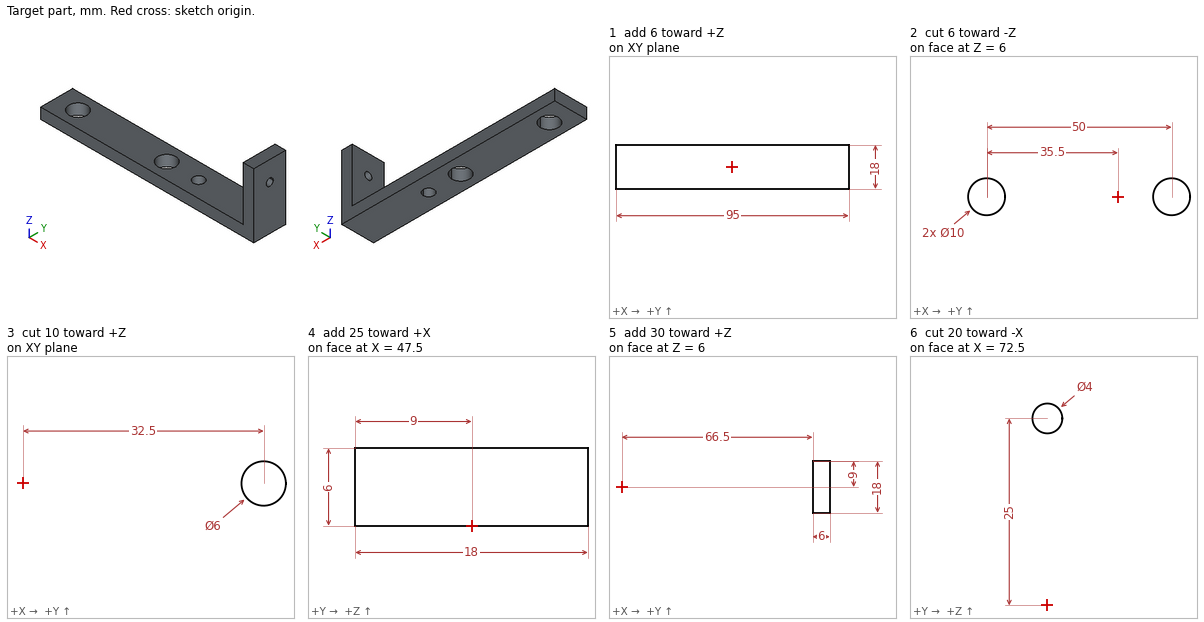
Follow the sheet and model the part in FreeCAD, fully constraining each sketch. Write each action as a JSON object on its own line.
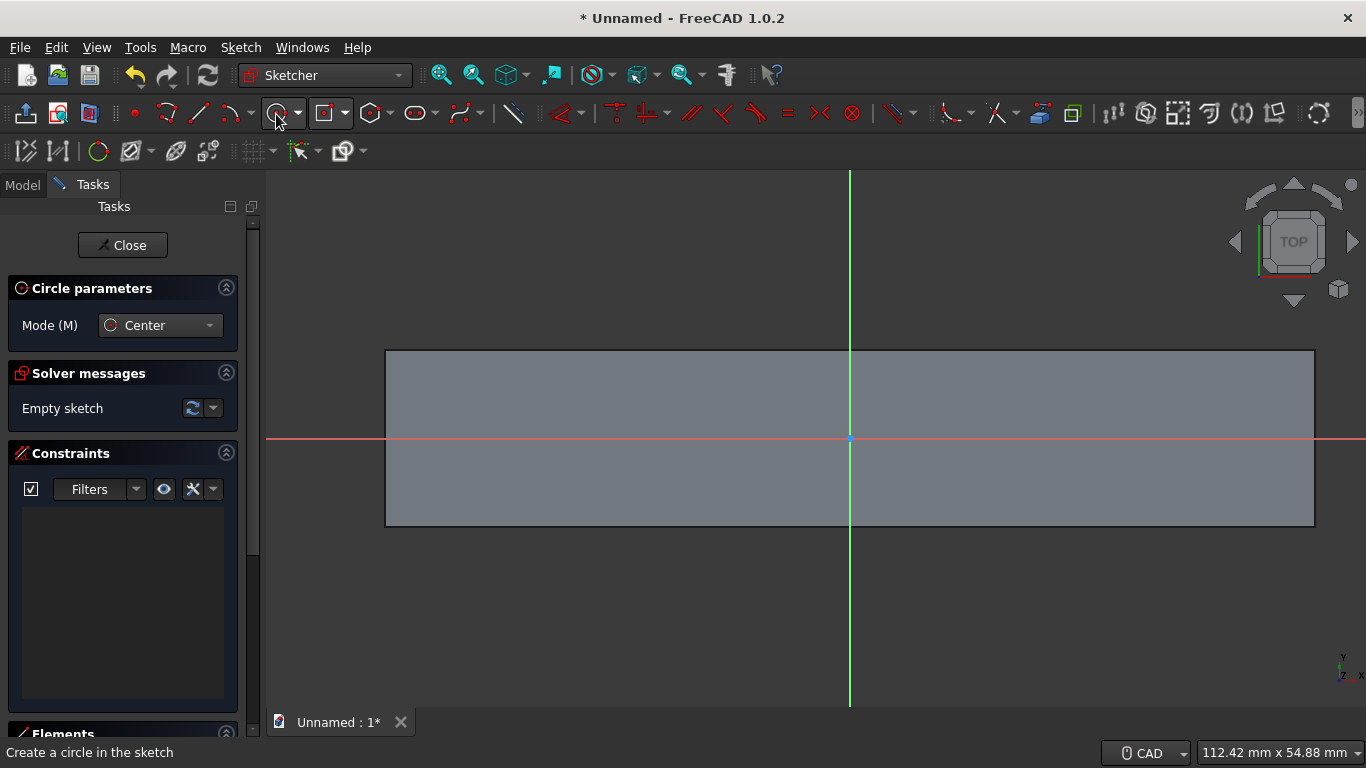
{"action": "left_click", "coordinate": [503, 438]}
{"action": "left_click", "coordinate": [537, 404]}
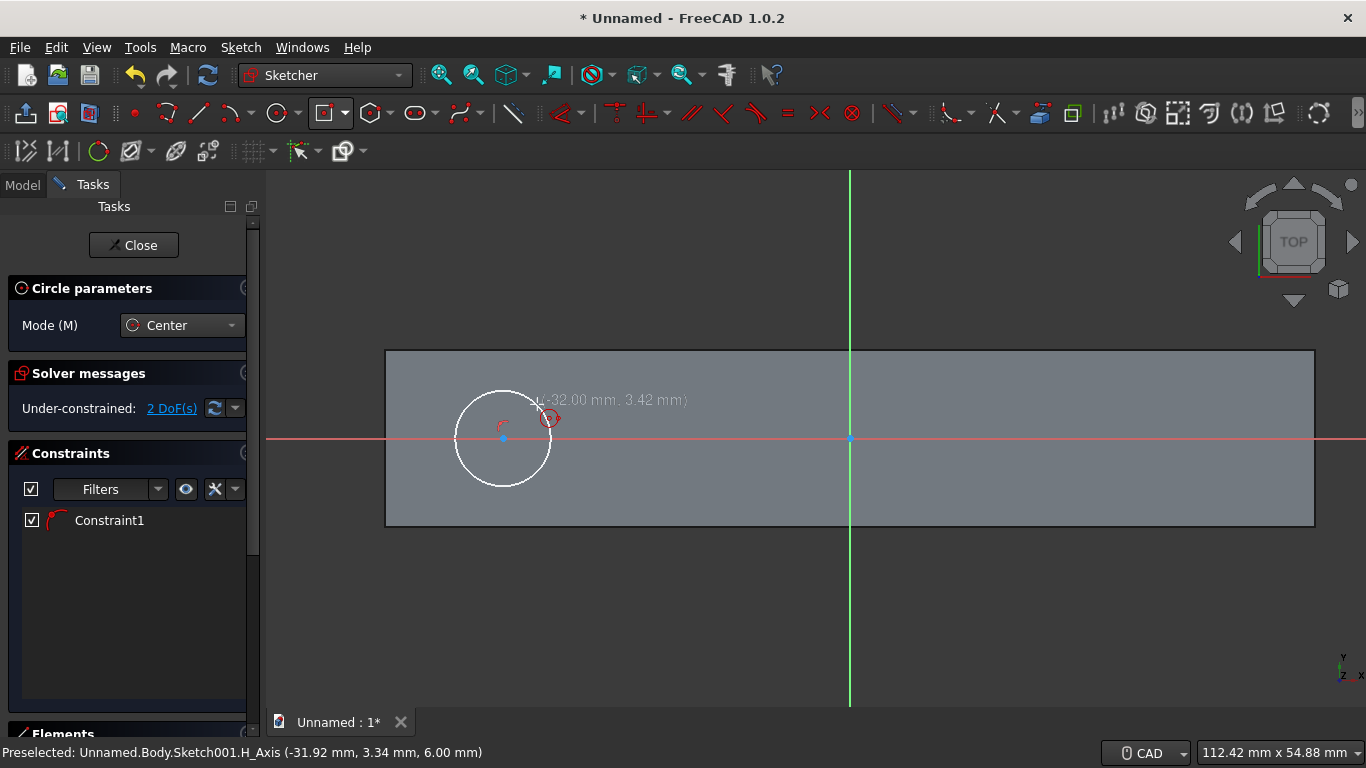
{"action": "left_click", "coordinate": [992, 438]}
{"action": "left_click", "coordinate": [1027, 404]}
{"action": "key", "text": "Escape"}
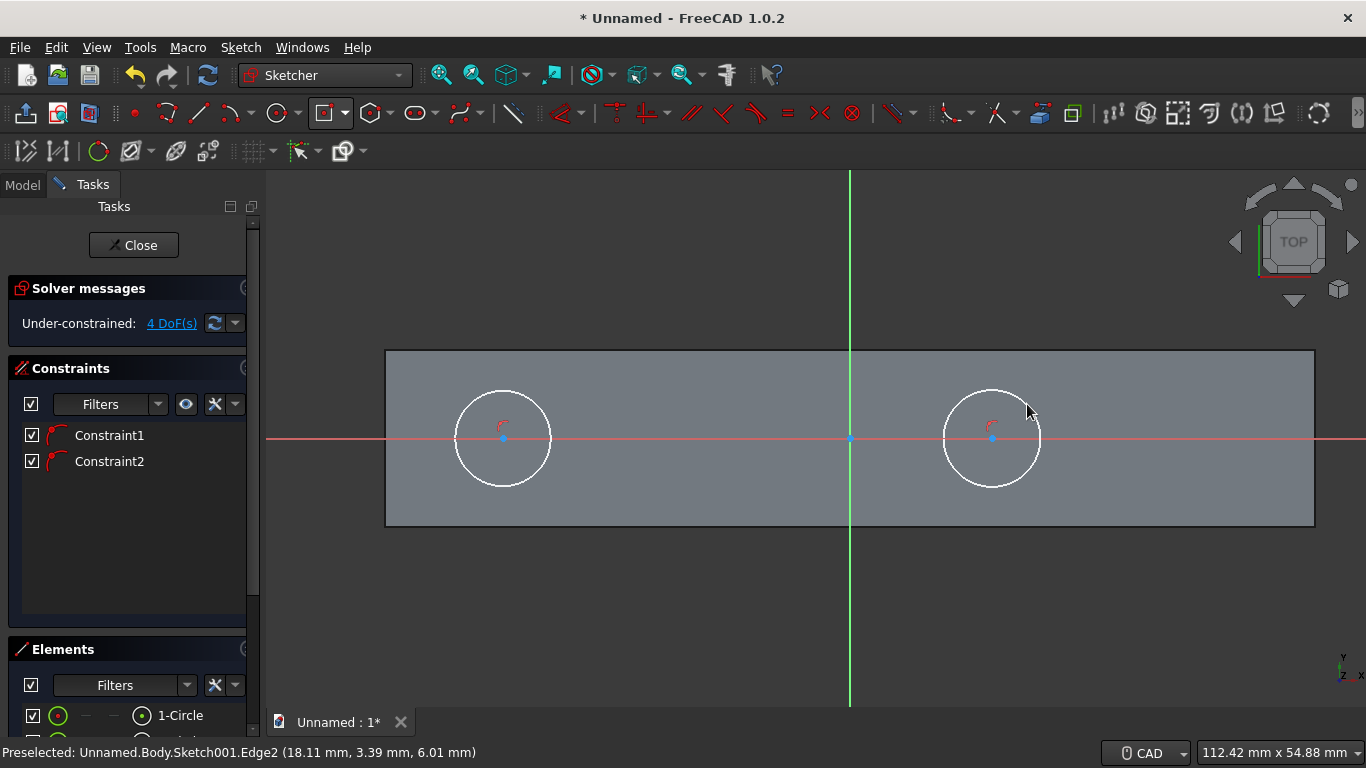
{"action": "left_click", "coordinate": [537, 405]}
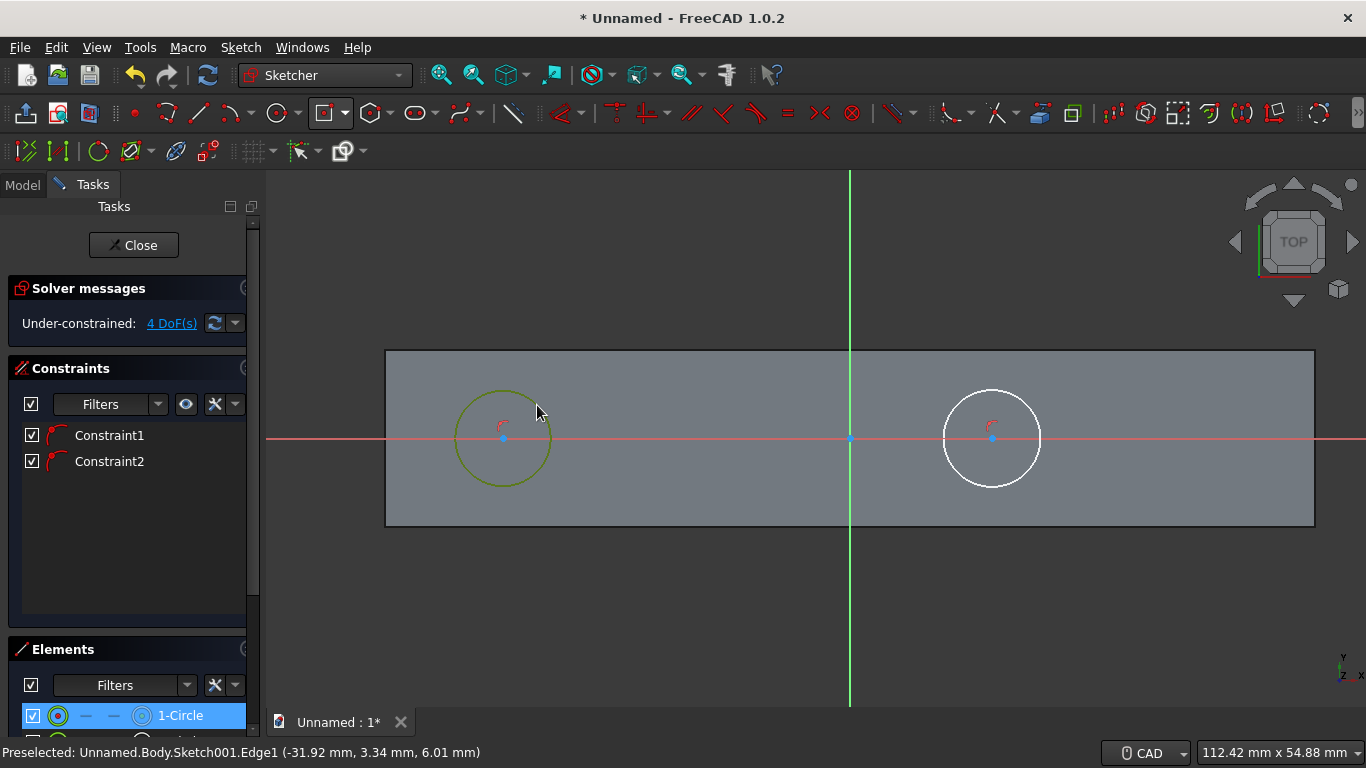
{"action": "left_click", "coordinate": [1026, 404]}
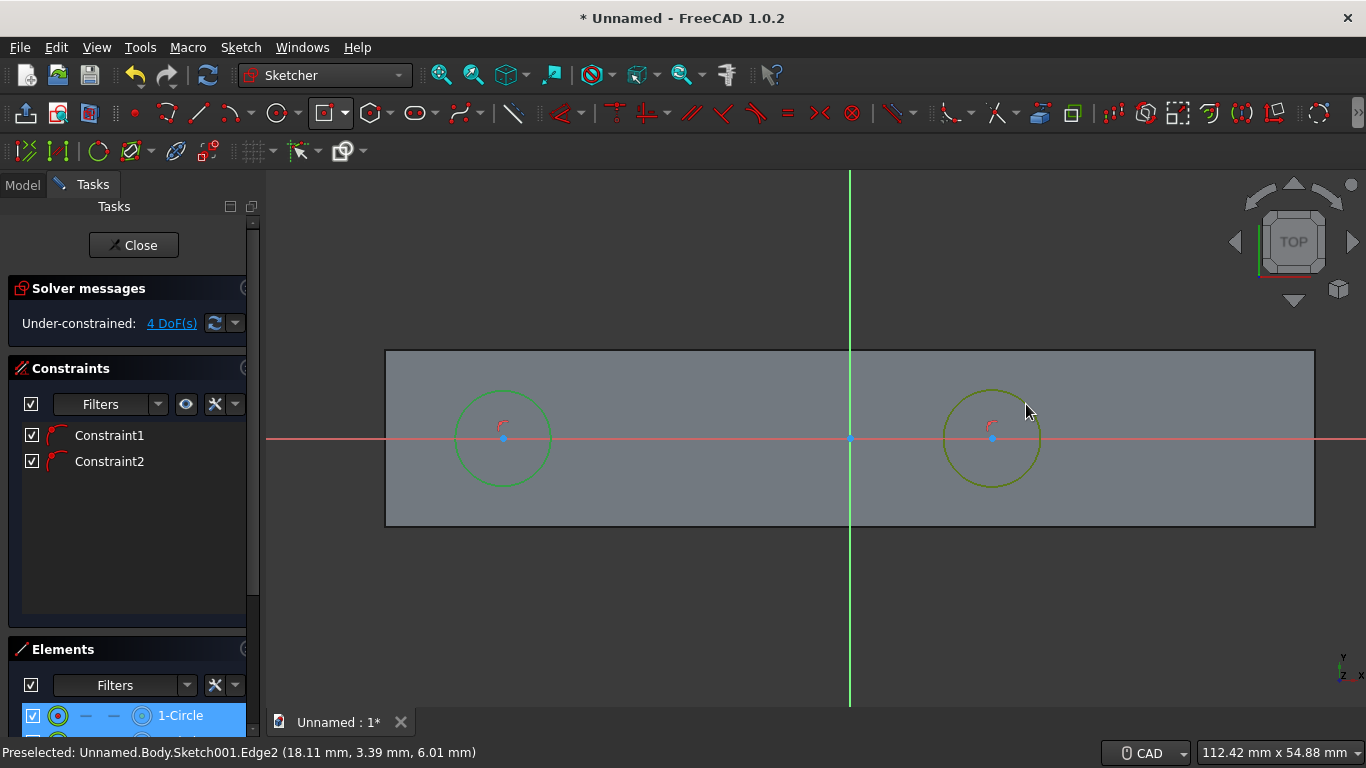
{"action": "left_click", "coordinate": [788, 114]}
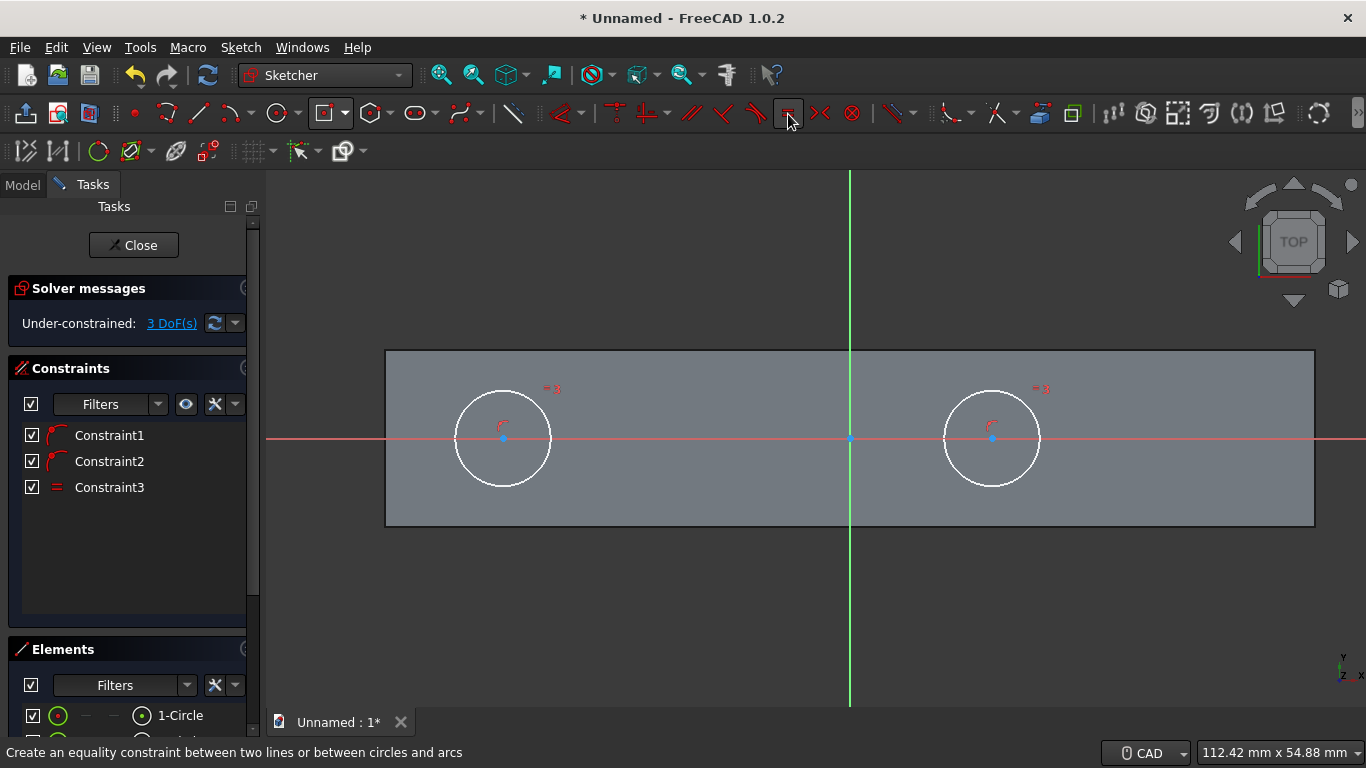
{"action": "left_click", "coordinate": [560, 114]}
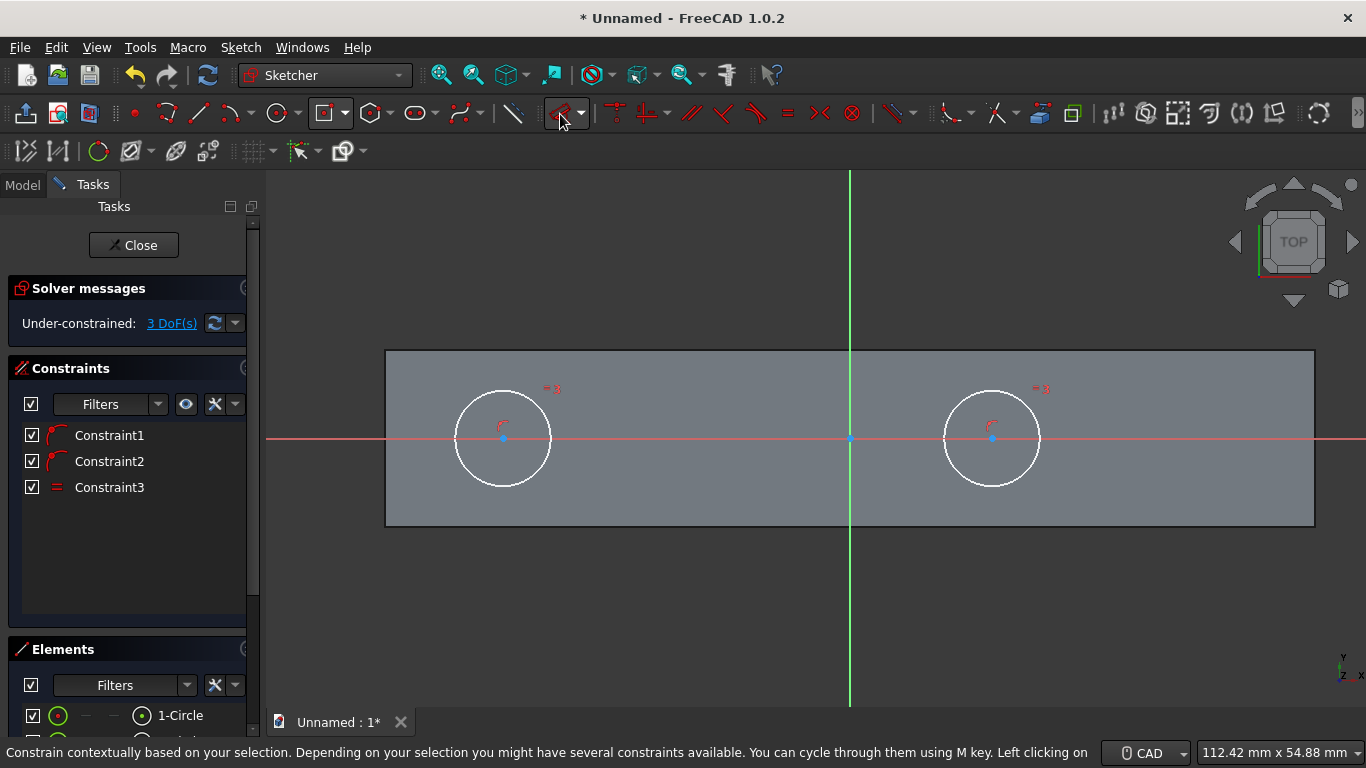
{"action": "left_click", "coordinate": [537, 405]}
{"action": "left_click", "coordinate": [560, 383]}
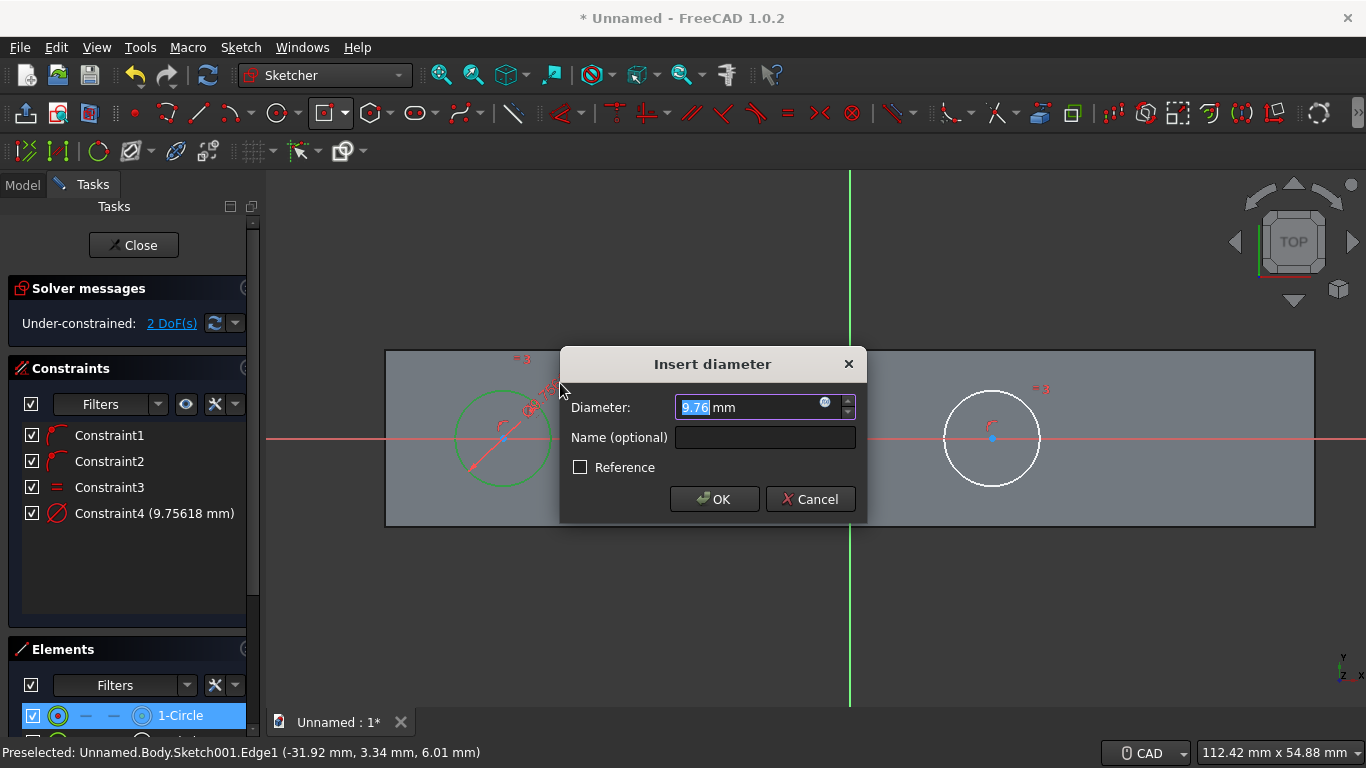
{"action": "type", "text": "10"}
{"action": "key", "text": "Return"}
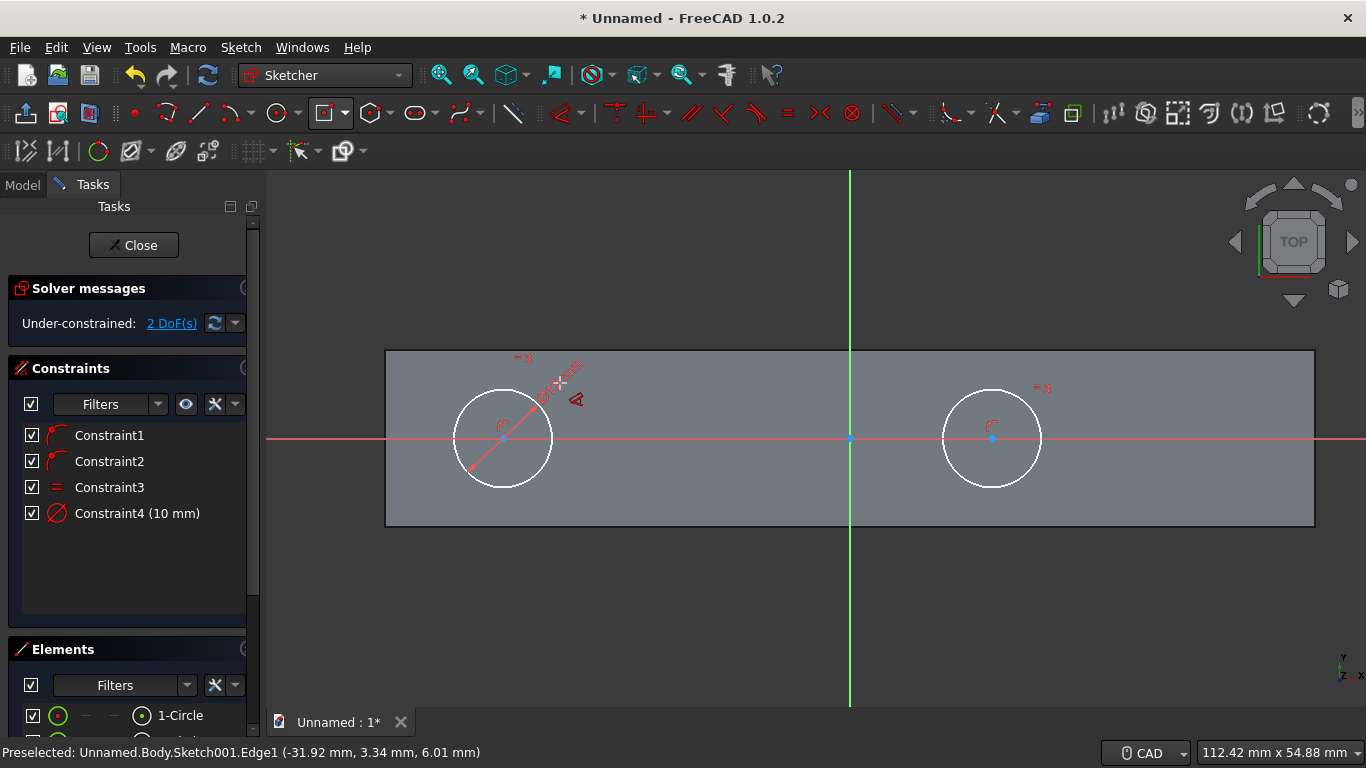
{"action": "left_click", "coordinate": [503, 438]}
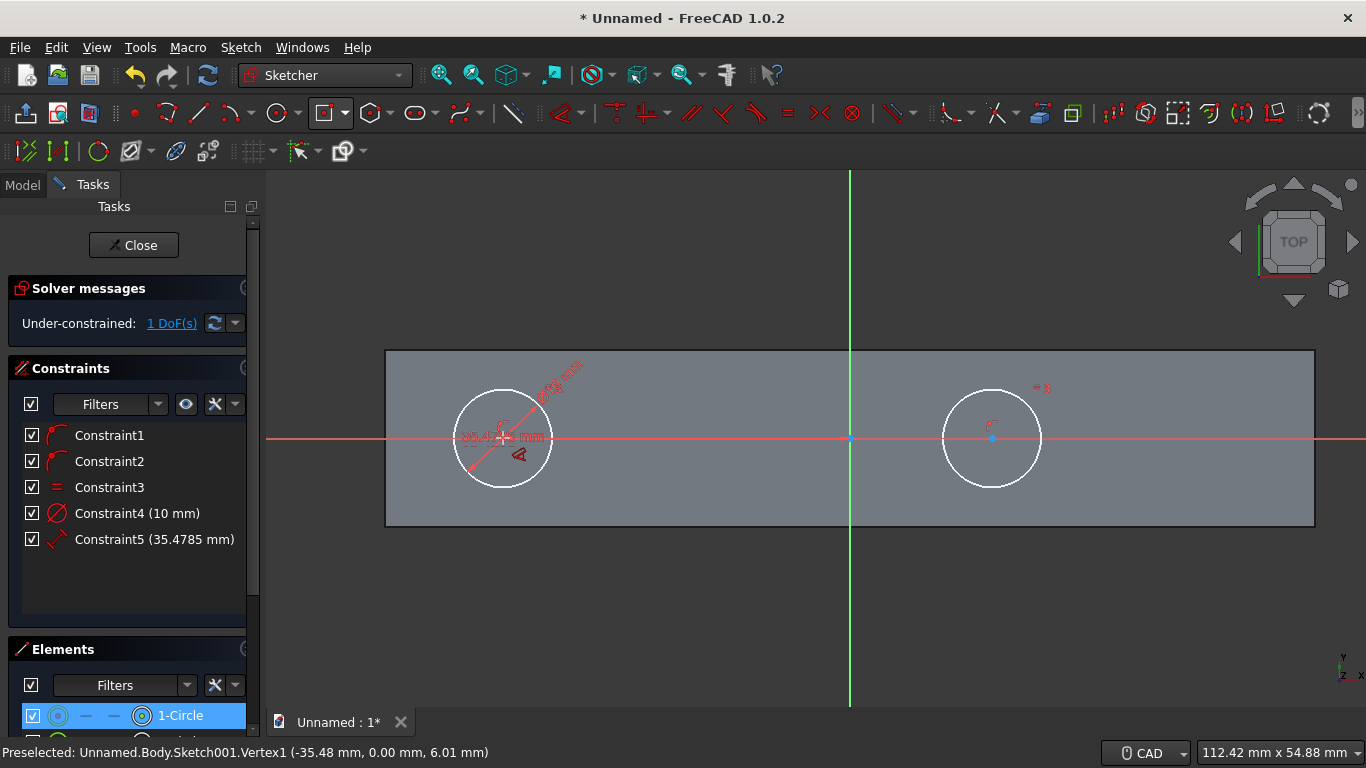
{"action": "left_click", "coordinate": [992, 438]}
{"action": "left_click", "coordinate": [748, 472]}